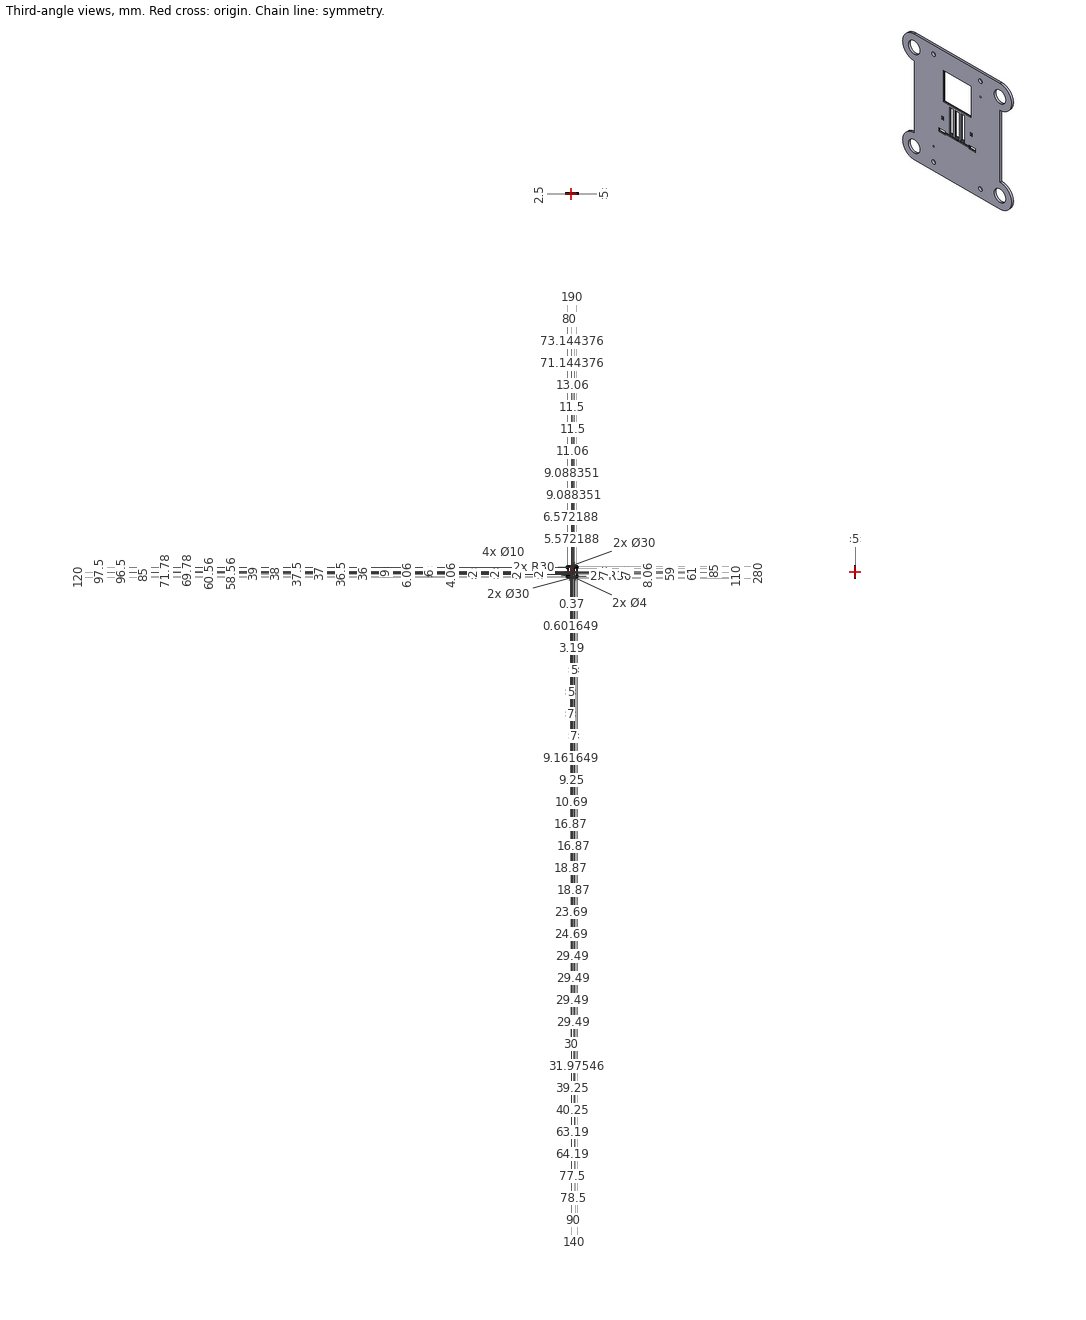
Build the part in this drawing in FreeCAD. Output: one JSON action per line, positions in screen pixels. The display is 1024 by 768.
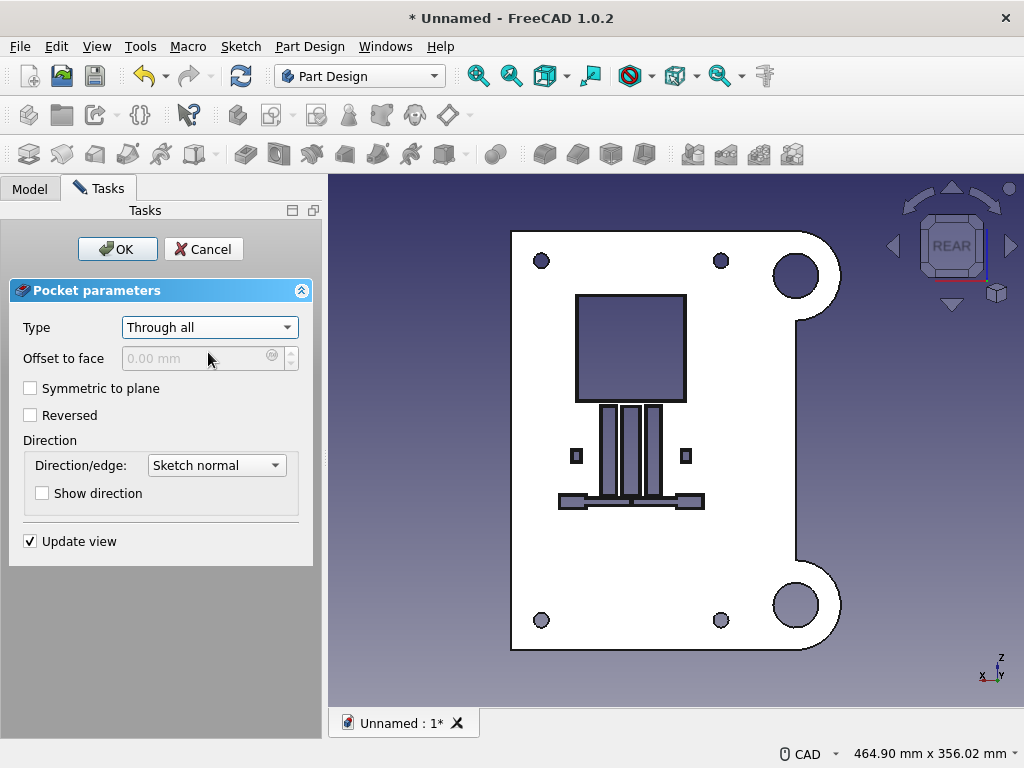
{"action": "left_click", "coordinate": [118, 249]}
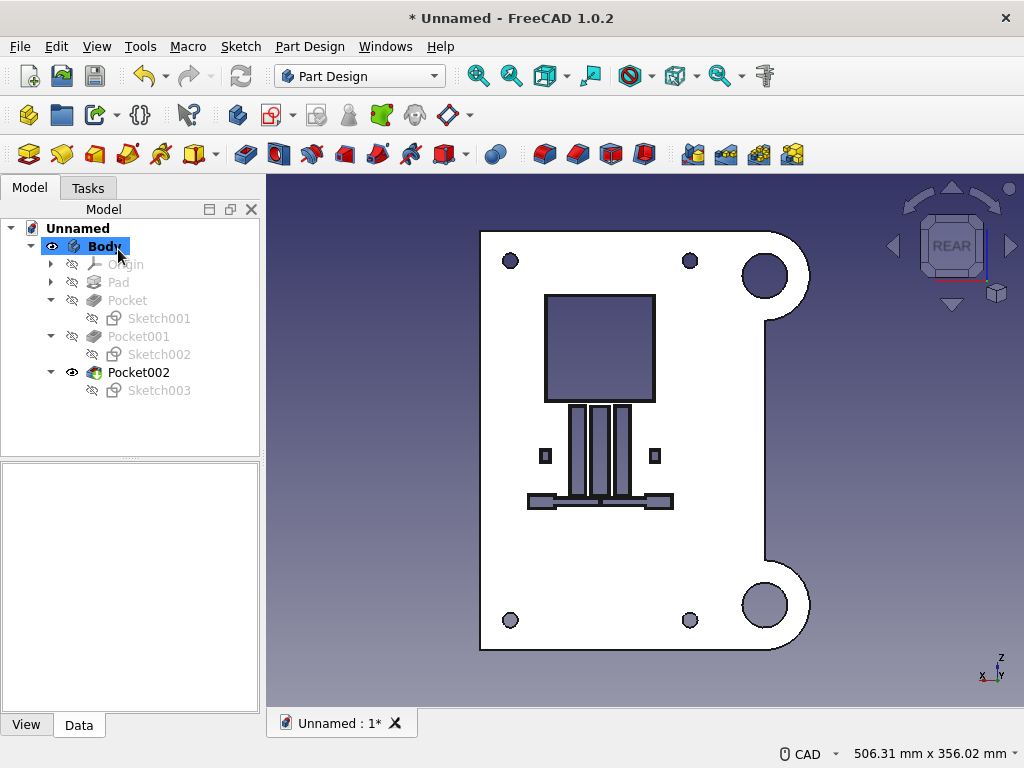
{"action": "left_click", "coordinate": [598, 559]}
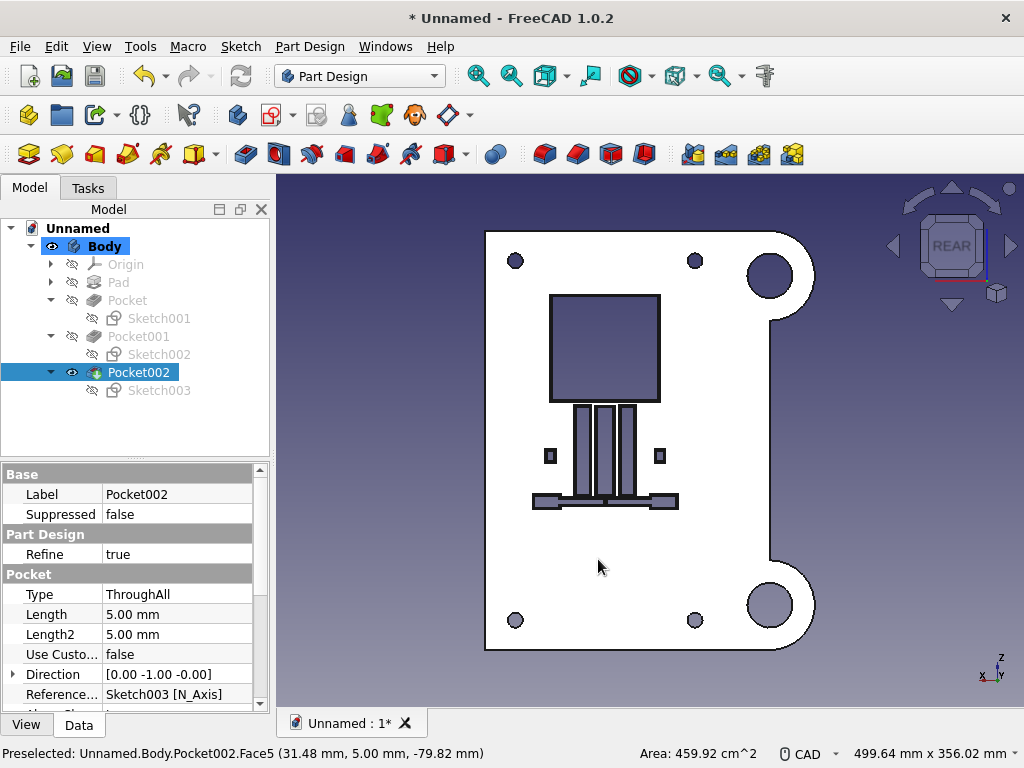
{"action": "left_click", "coordinate": [270, 116]}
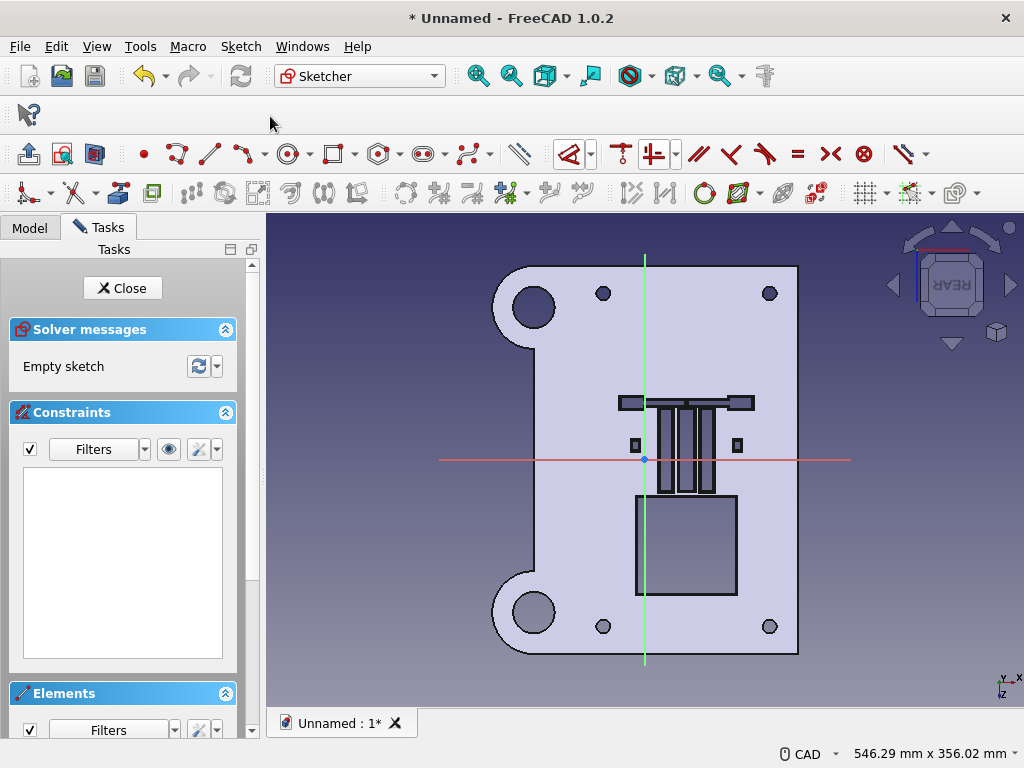
{"action": "scroll", "coordinate": [294, 460], "scroll_direction": "down", "scroll_amount": 1}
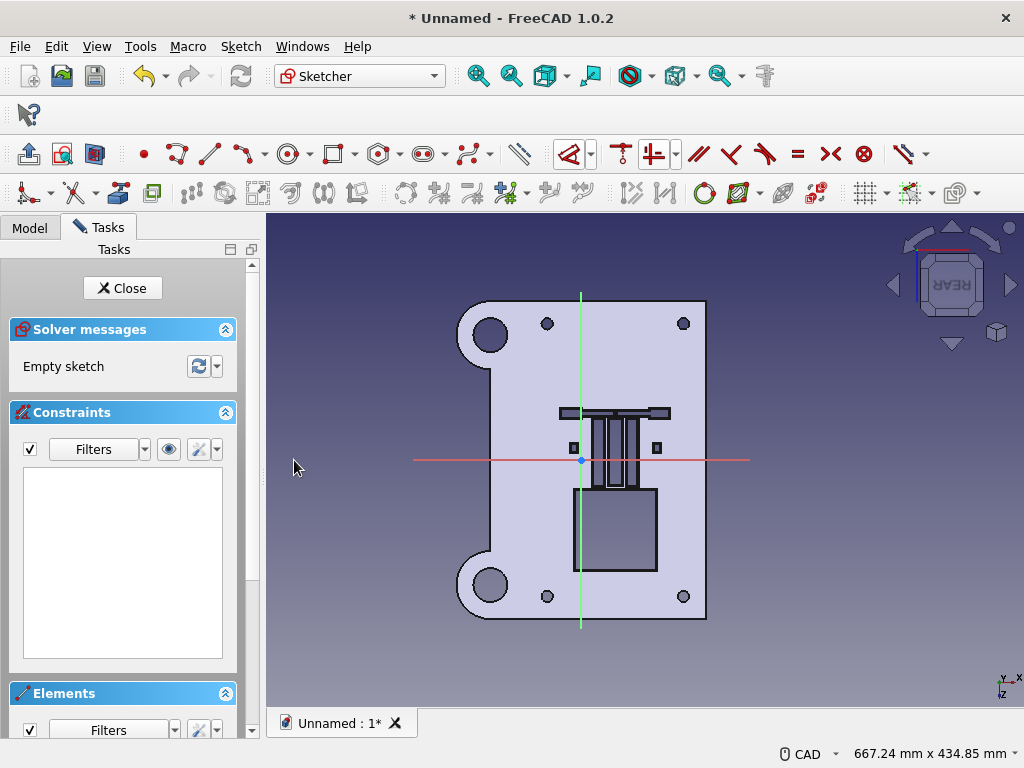
{"action": "left_click", "coordinate": [177, 154]}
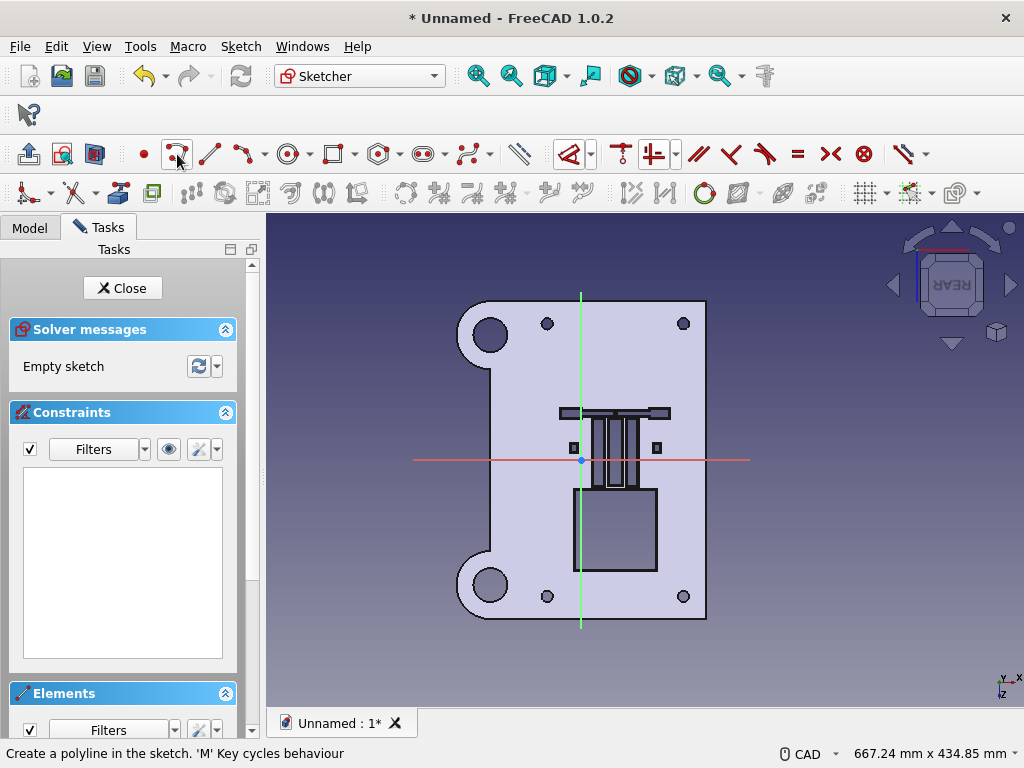
{"action": "left_click", "coordinate": [740, 301]}
{"action": "left_click", "coordinate": [704, 301]}
{"action": "left_click", "coordinate": [704, 619]}
{"action": "left_click", "coordinate": [740, 619]}
{"action": "right_click", "coordinate": [740, 619]}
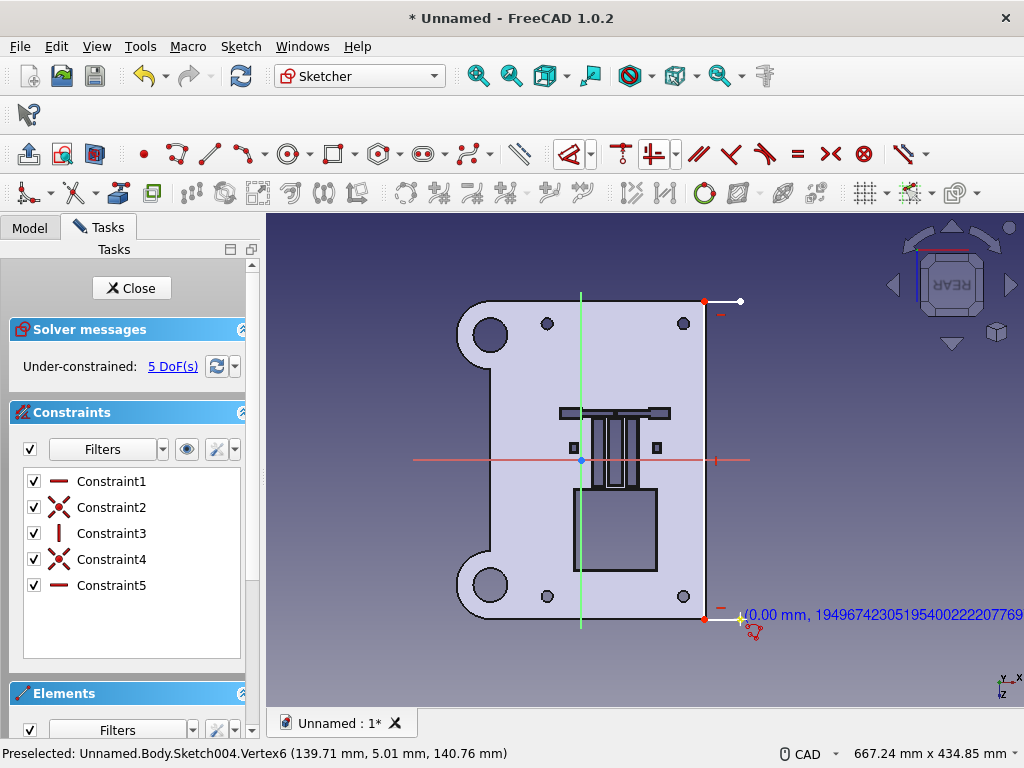
{"action": "left_click", "coordinate": [210, 154]}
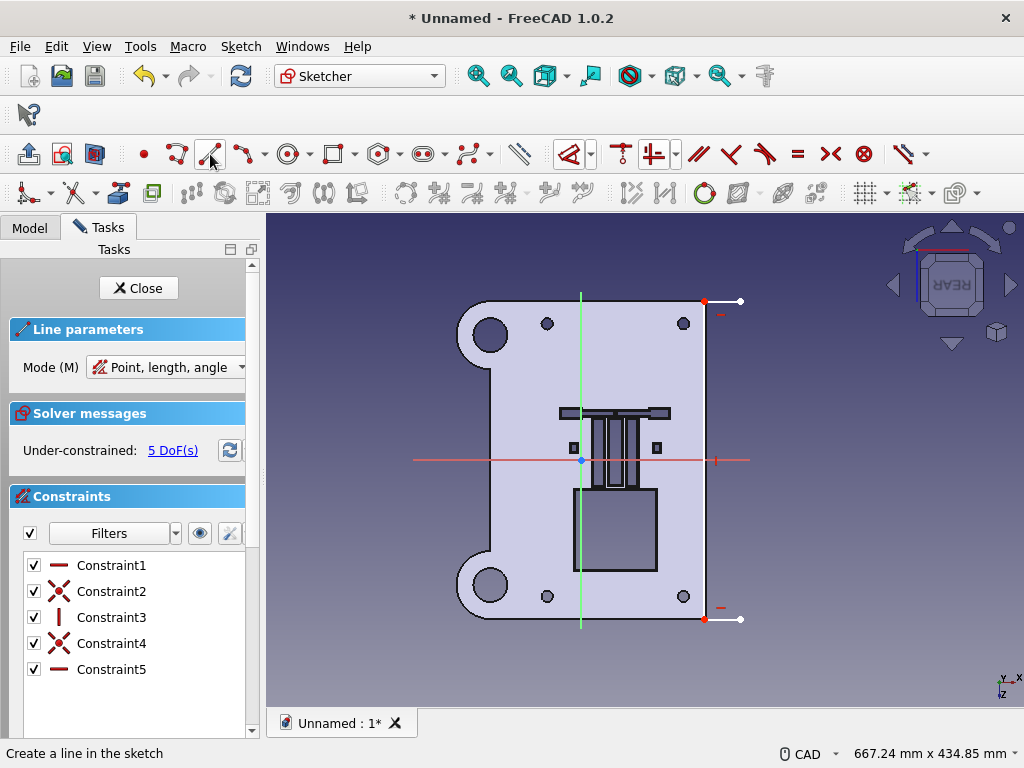
{"action": "left_click", "coordinate": [740, 551]}
{"action": "left_click", "coordinate": [740, 369]}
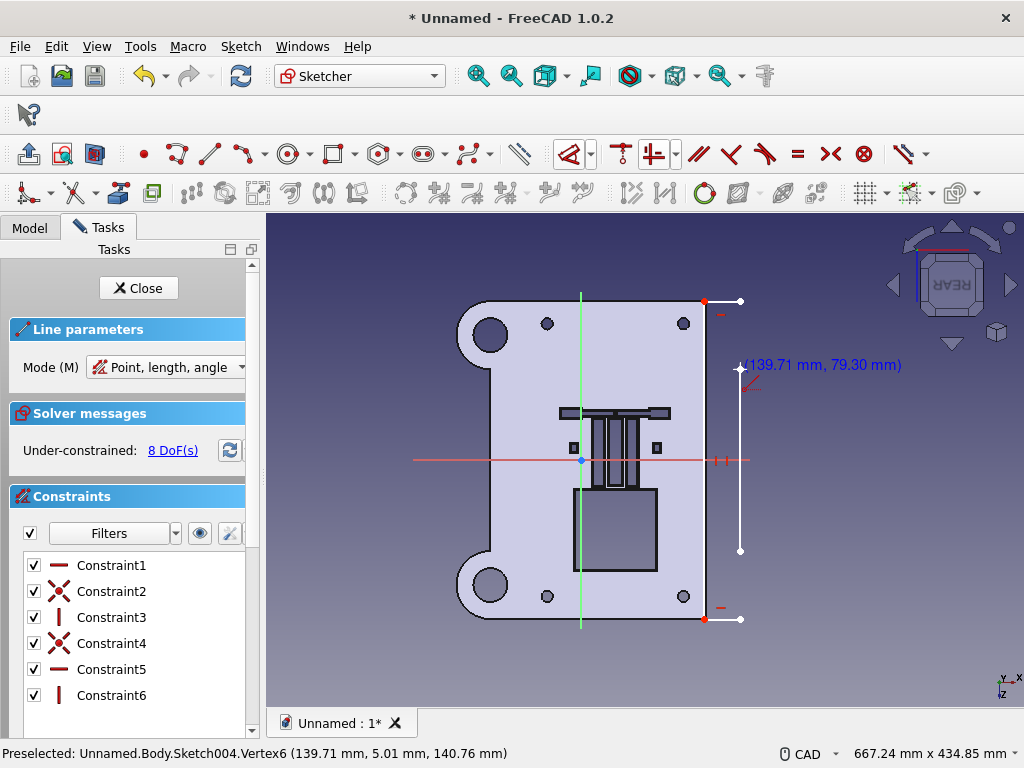
{"action": "left_click", "coordinate": [242, 154]}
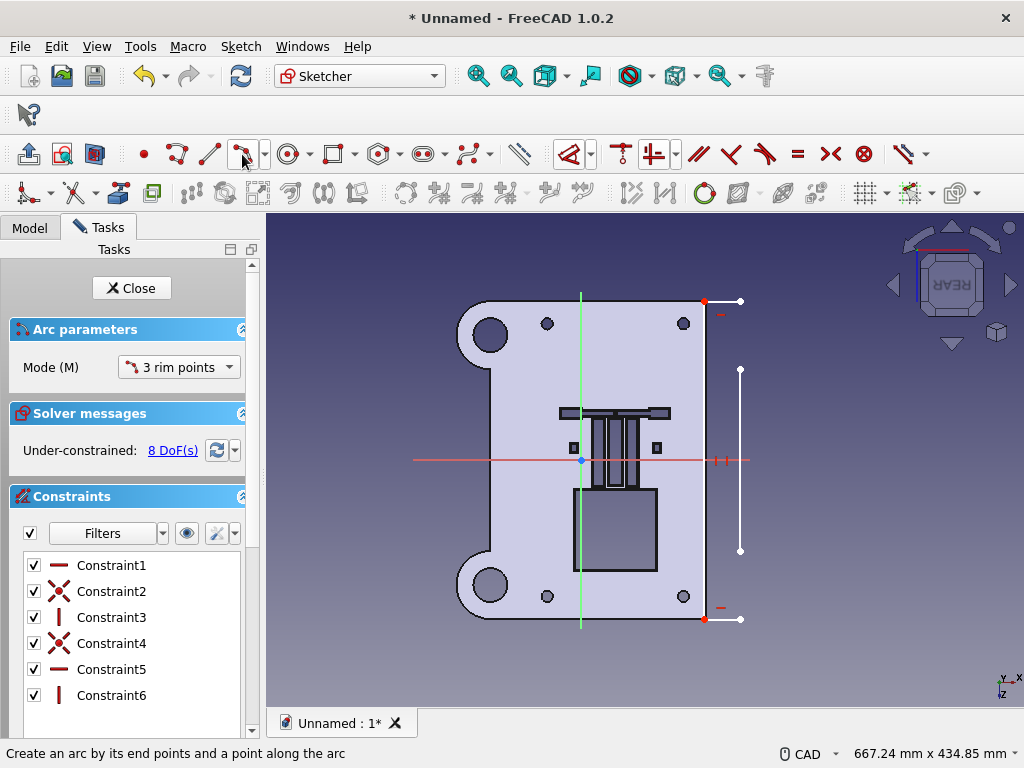
{"action": "left_click", "coordinate": [740, 620]}
{"action": "left_click", "coordinate": [740, 552]}
{"action": "left_click", "coordinate": [774, 585]}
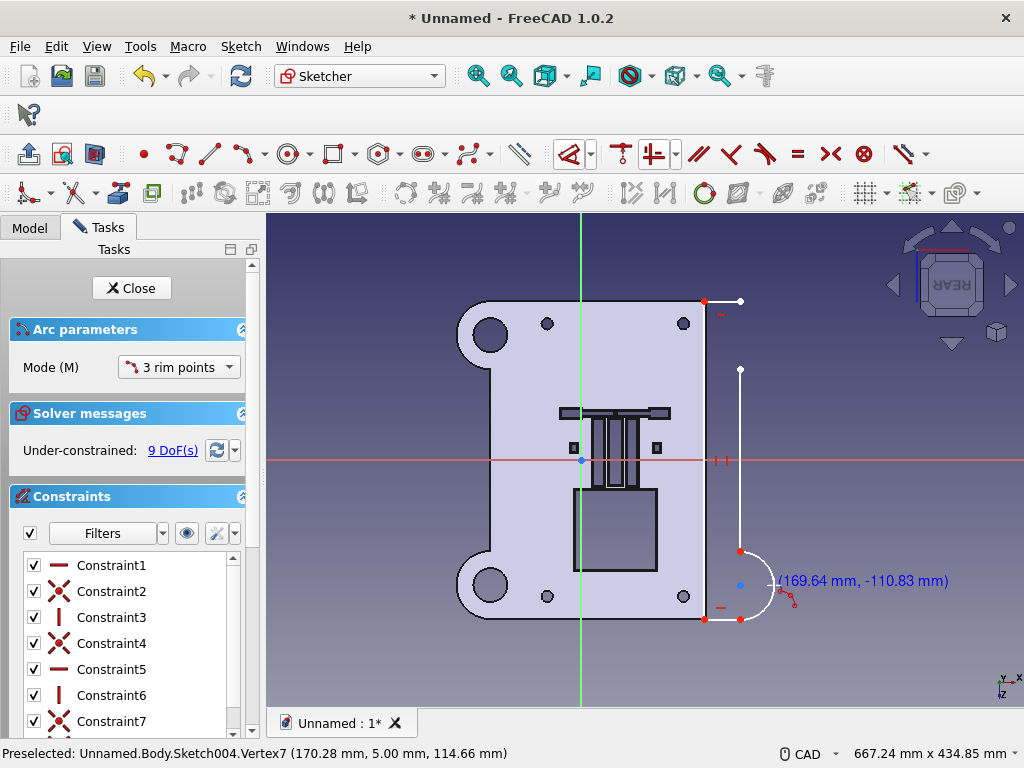
{"action": "left_click", "coordinate": [740, 370]}
{"action": "left_click", "coordinate": [740, 302]}
{"action": "left_click", "coordinate": [774, 335]}
{"action": "key", "text": "Escape"}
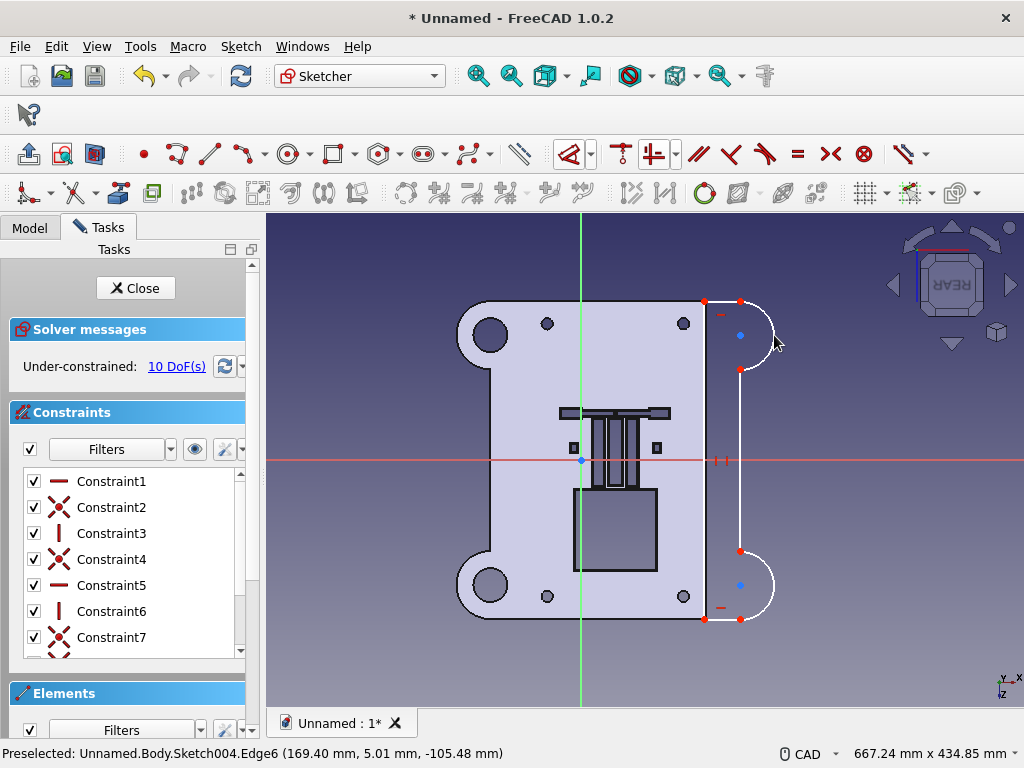
{"action": "scroll", "coordinate": [729, 302], "scroll_direction": "up", "scroll_amount": 2}